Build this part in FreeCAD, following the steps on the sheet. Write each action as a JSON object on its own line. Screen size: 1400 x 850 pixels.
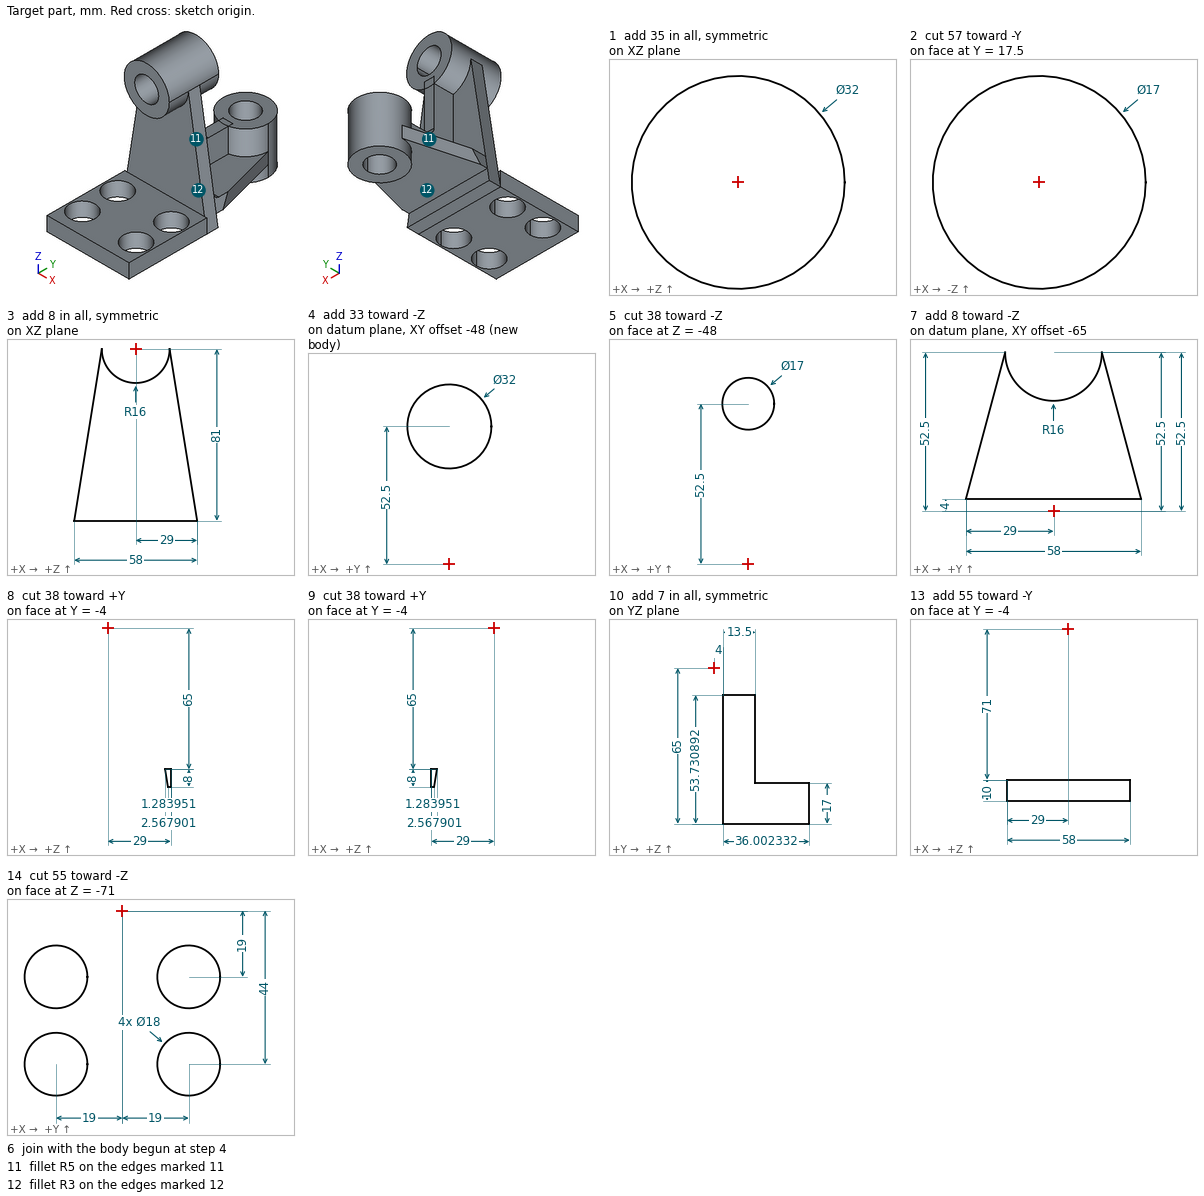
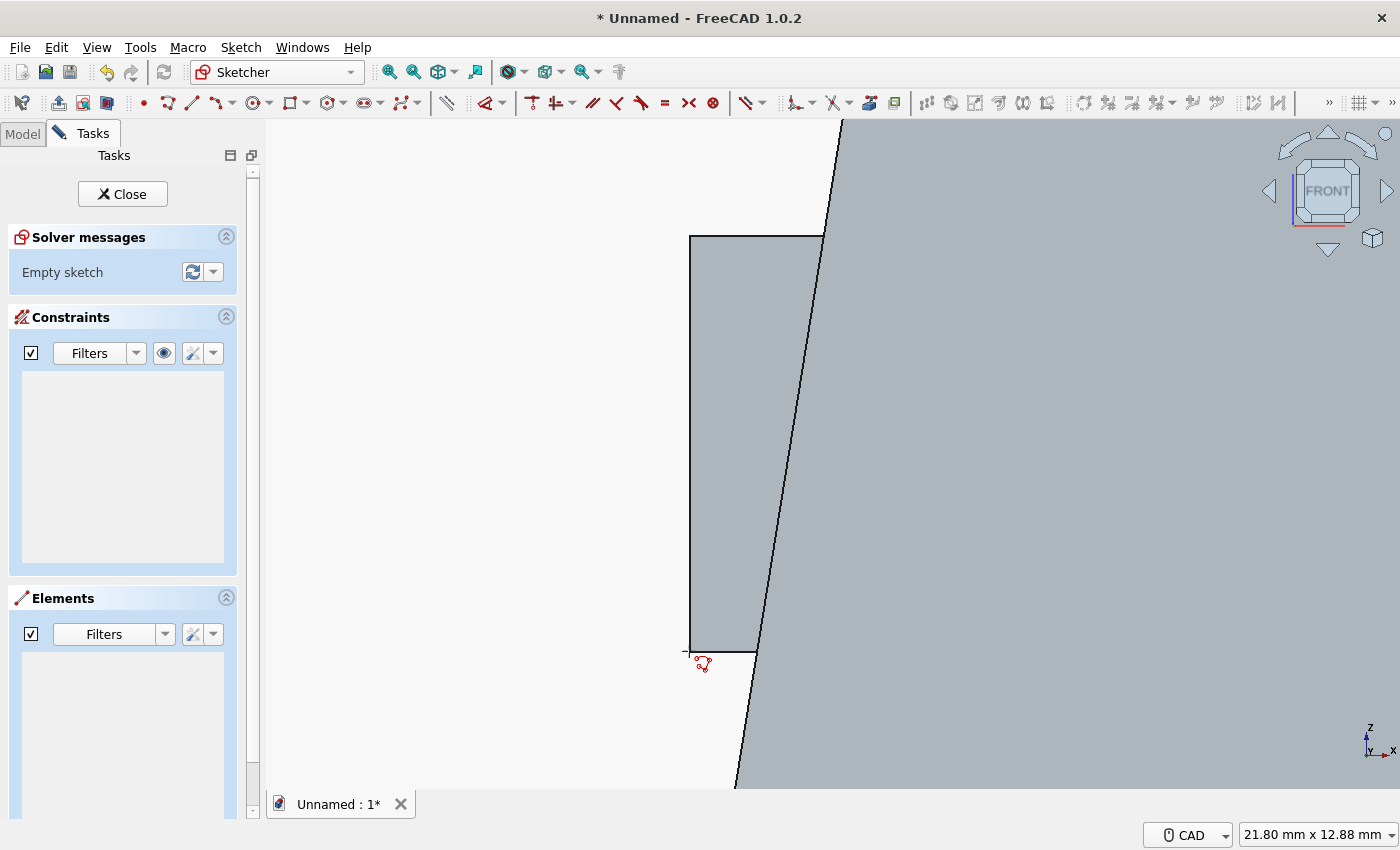
{"action": "left_click", "coordinate": [824, 236]}
{"action": "left_click", "coordinate": [690, 236]}
{"action": "left_click", "coordinate": [690, 652]}
{"action": "left_click", "coordinate": [757, 652]}
{"action": "left_click", "coordinate": [824, 237]}
{"action": "key", "text": "Escape"}
{"action": "key", "text": "Escape"}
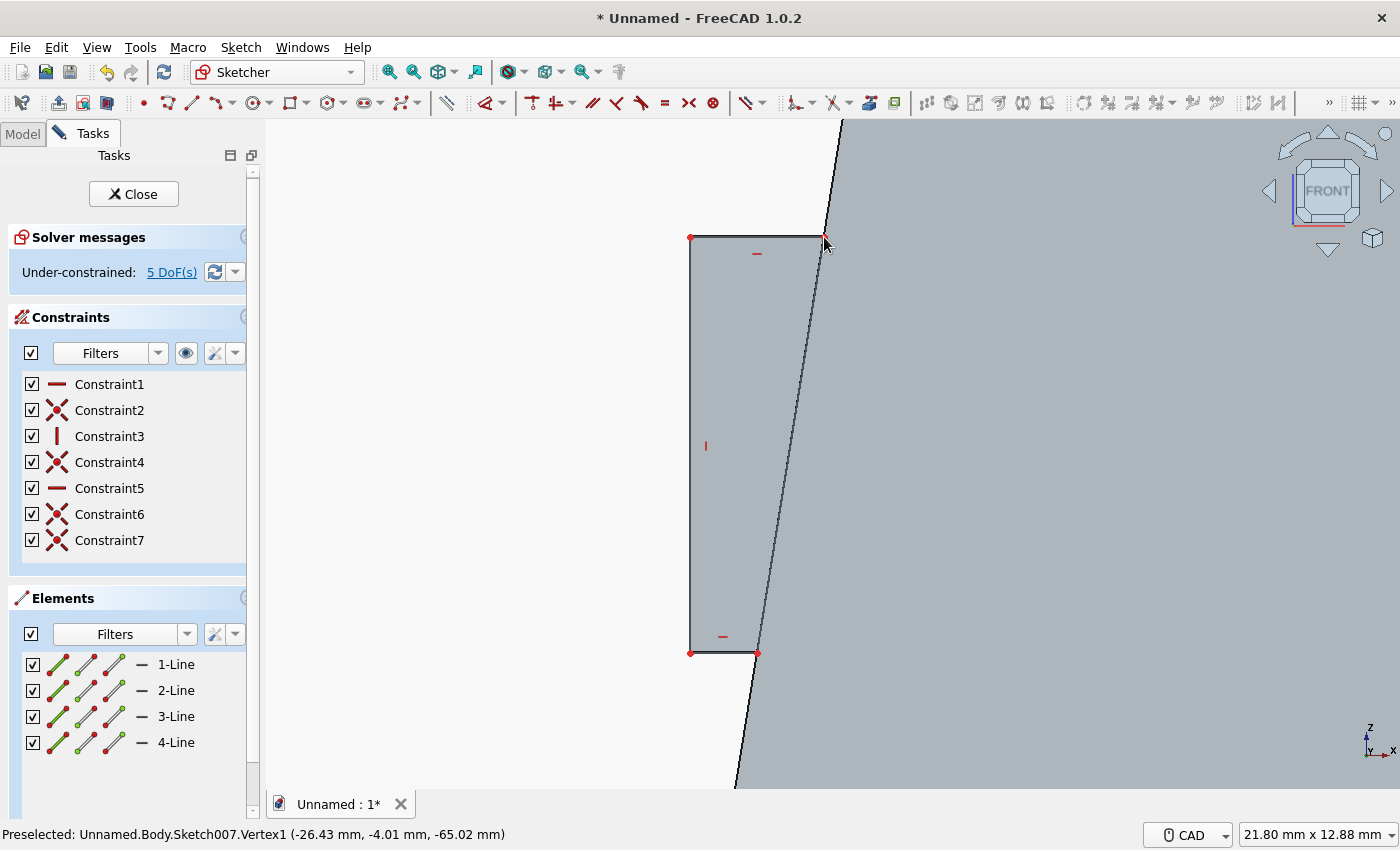
{"action": "key", "text": "d"}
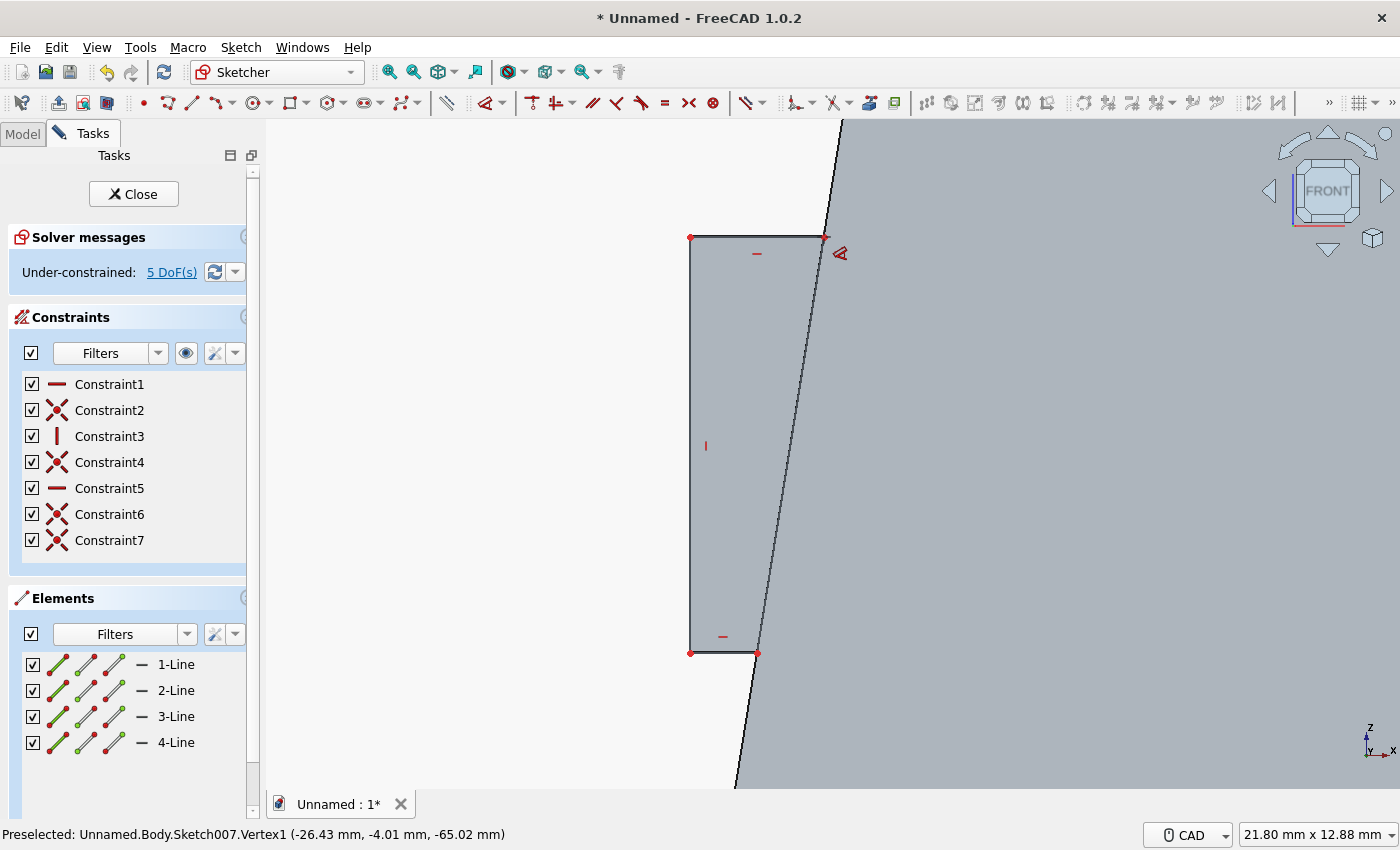
{"action": "left_click", "coordinate": [690, 362]}
{"action": "left_click", "coordinate": [656, 445]}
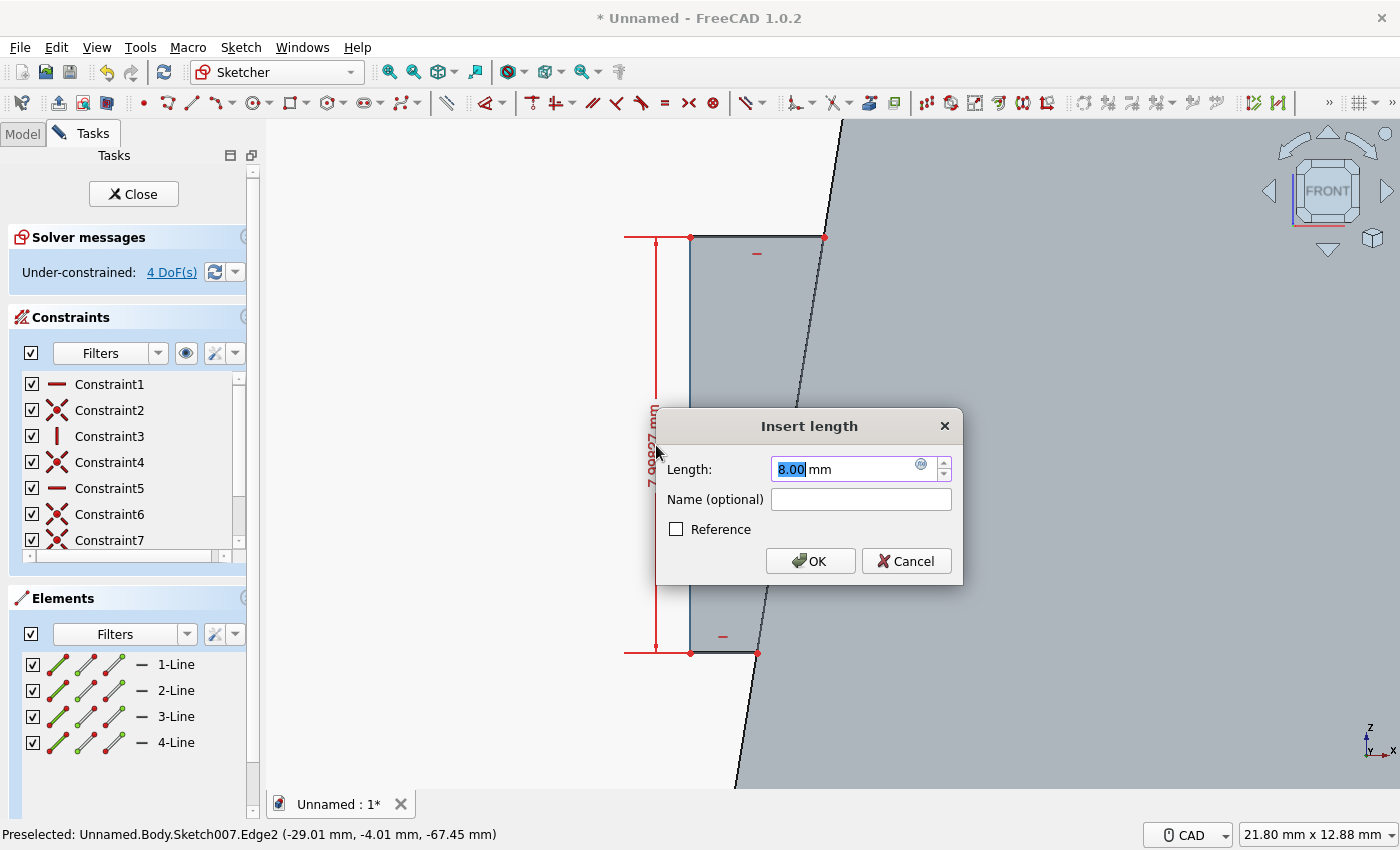
{"action": "type", "text": "8"}
{"action": "key", "text": "Return"}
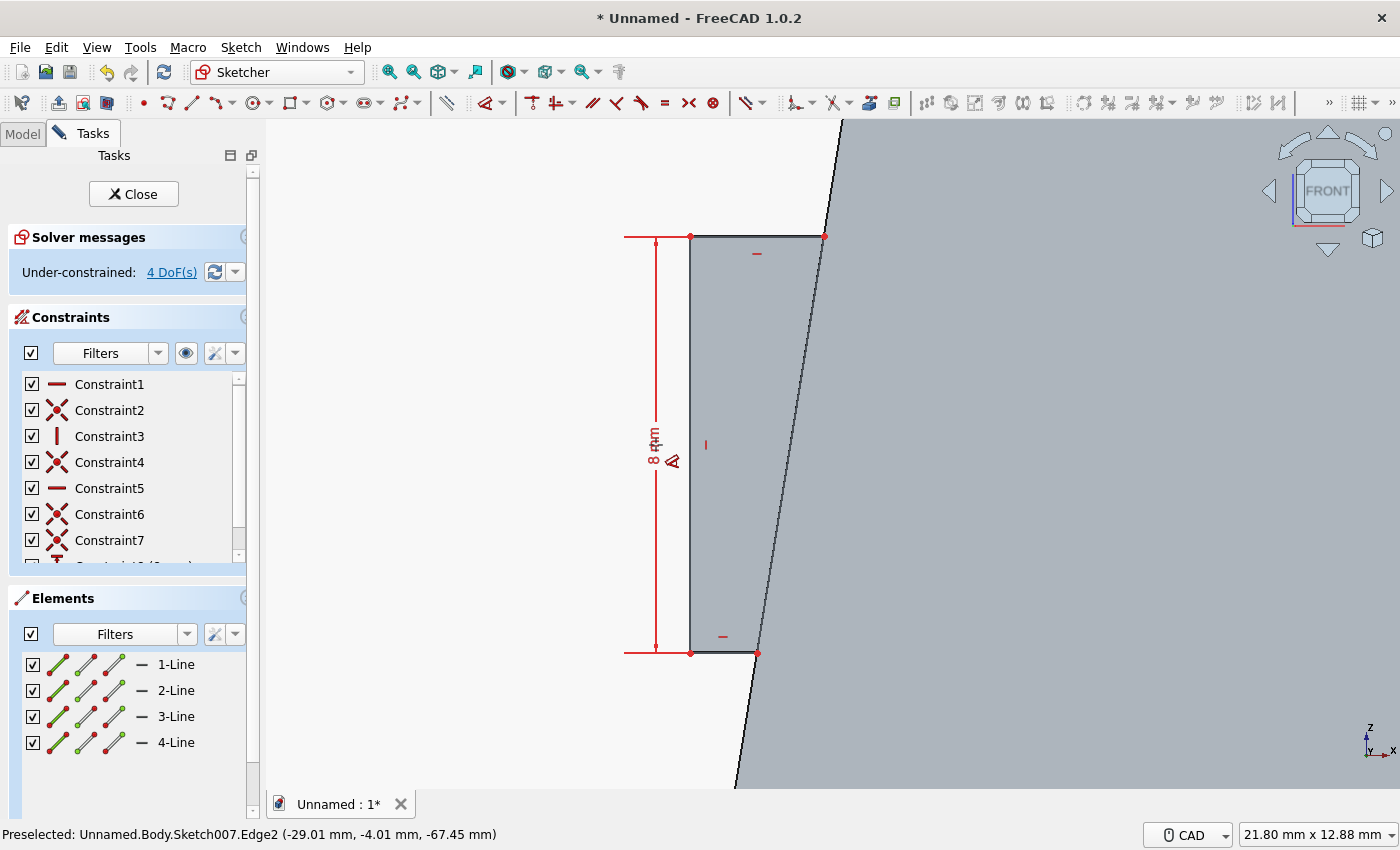
{"action": "left_click", "coordinate": [824, 237]}
{"action": "left_click", "coordinate": [790, 192]}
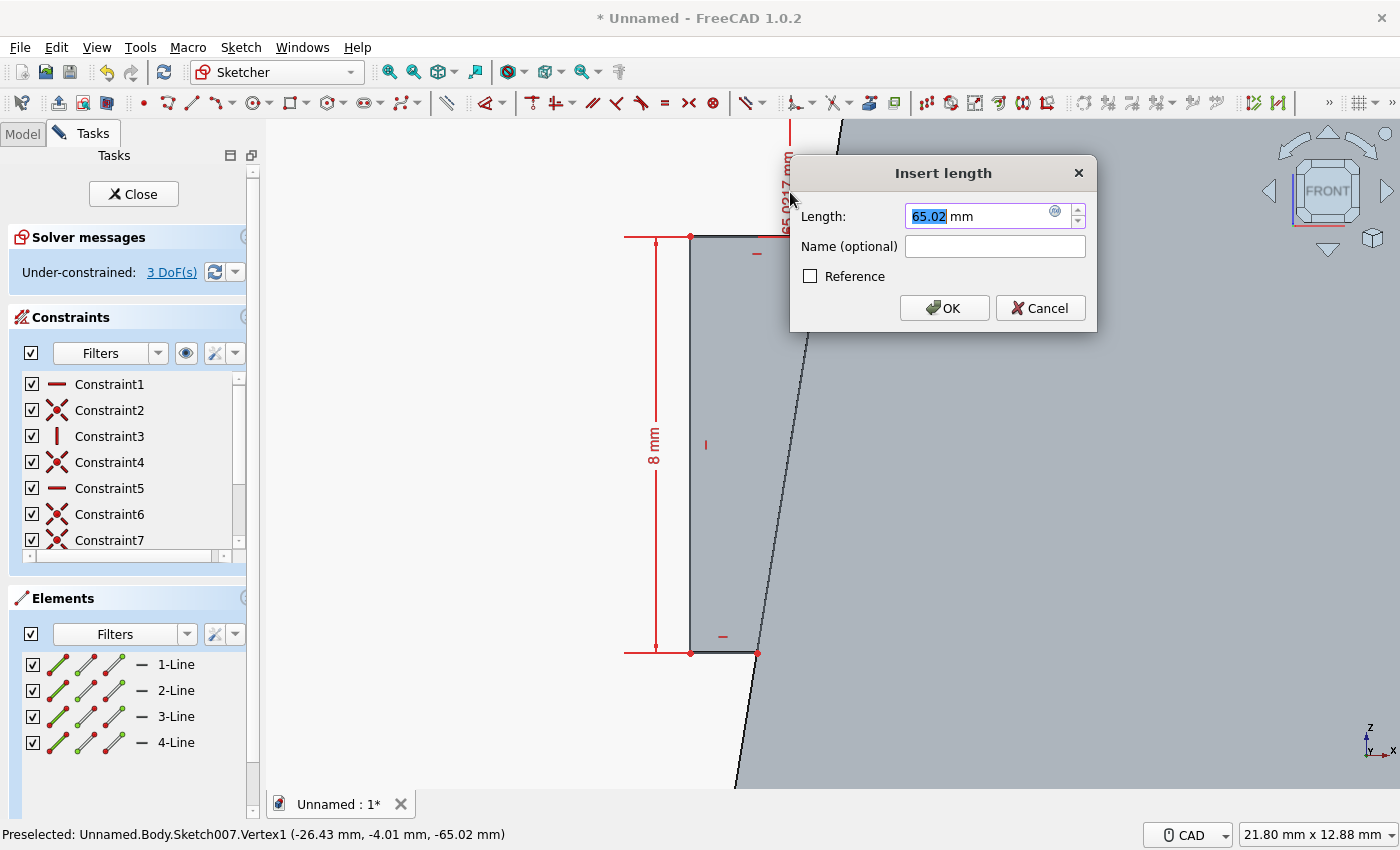
{"action": "type", "text": "65"}
{"action": "key", "text": "Return"}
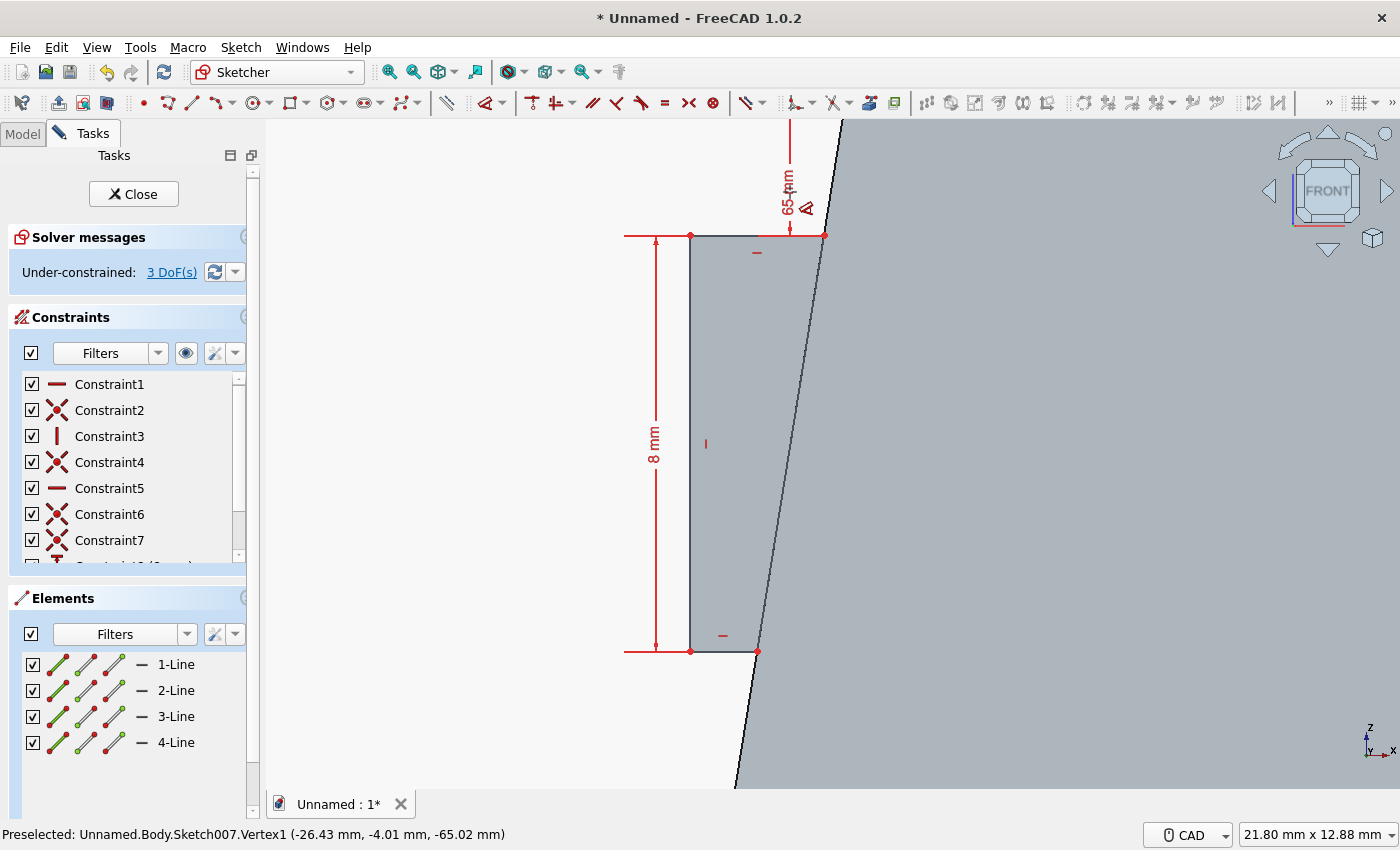
{"action": "left_click", "coordinate": [690, 236]}
{"action": "left_click", "coordinate": [962, 270]}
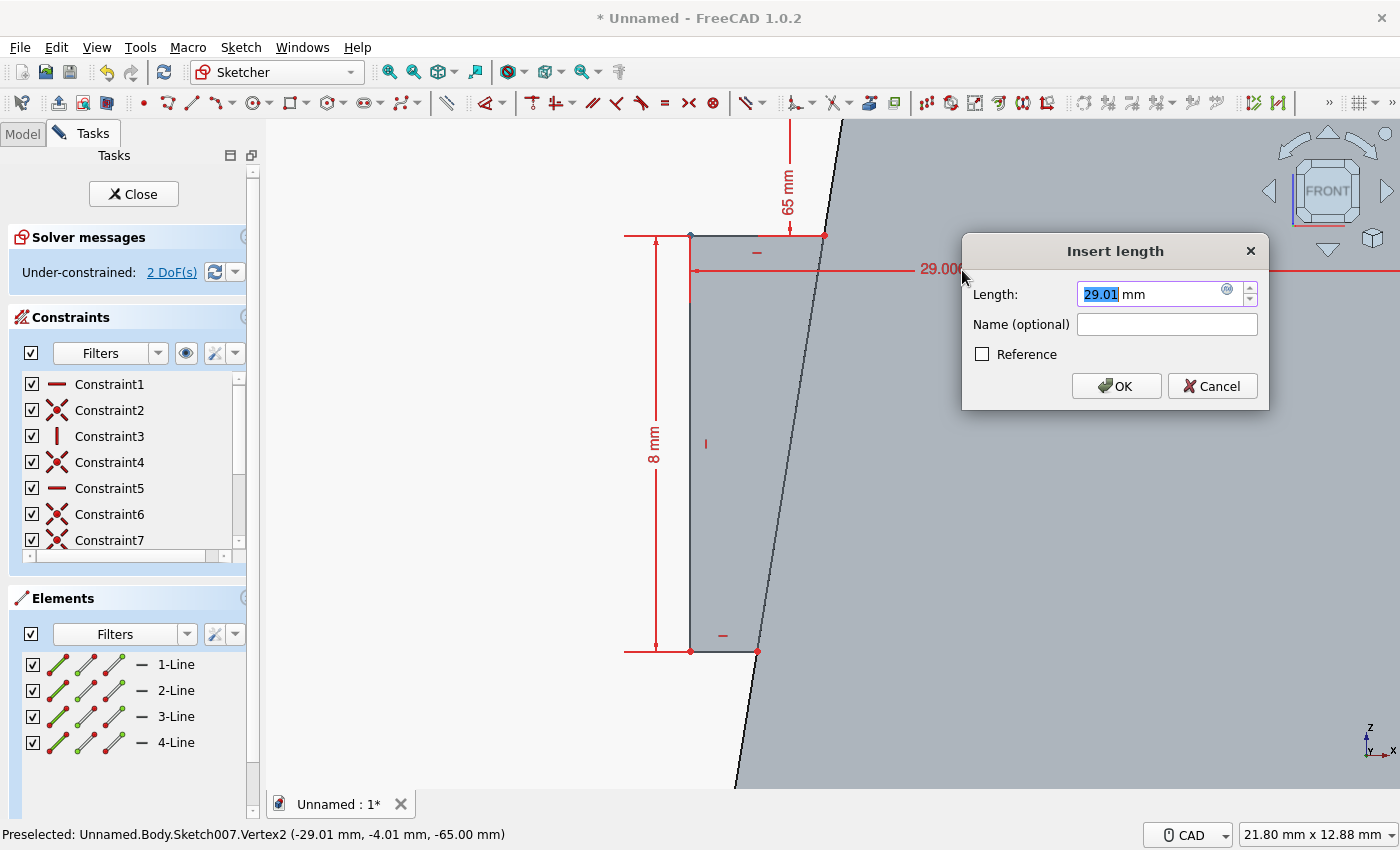
{"action": "type", "text": "29"}
{"action": "key", "text": "Return"}